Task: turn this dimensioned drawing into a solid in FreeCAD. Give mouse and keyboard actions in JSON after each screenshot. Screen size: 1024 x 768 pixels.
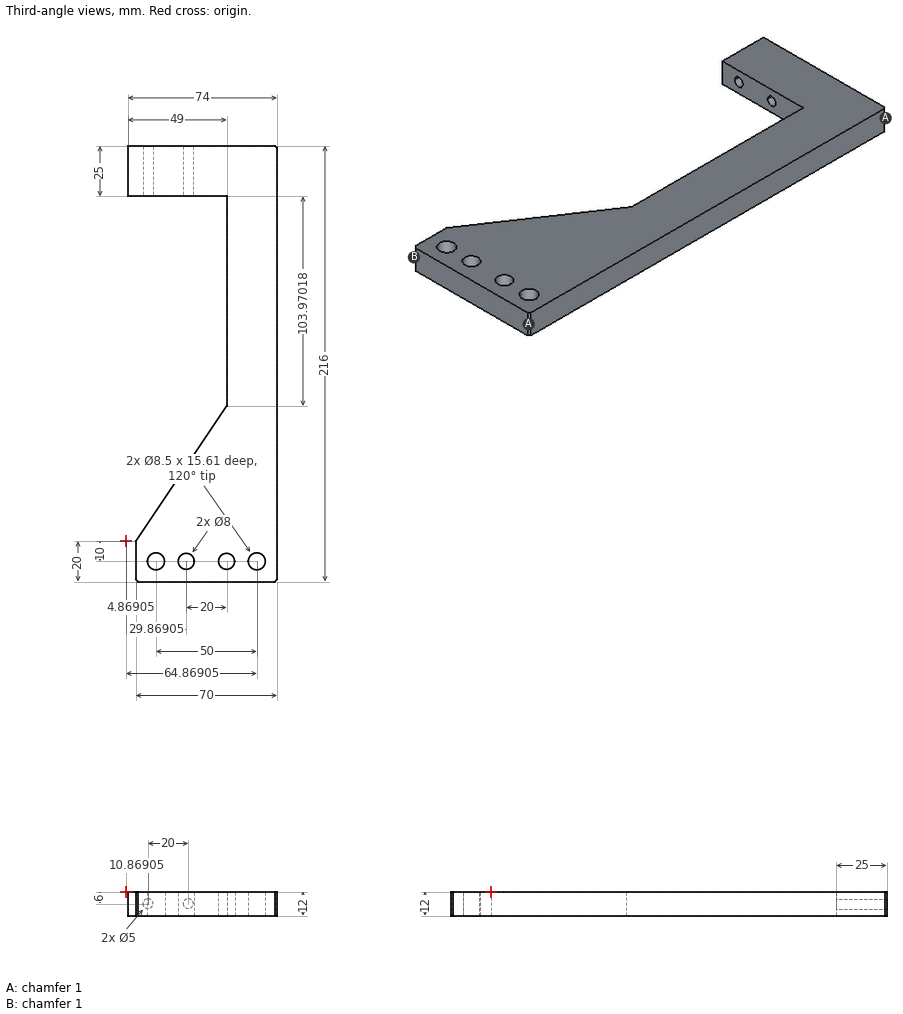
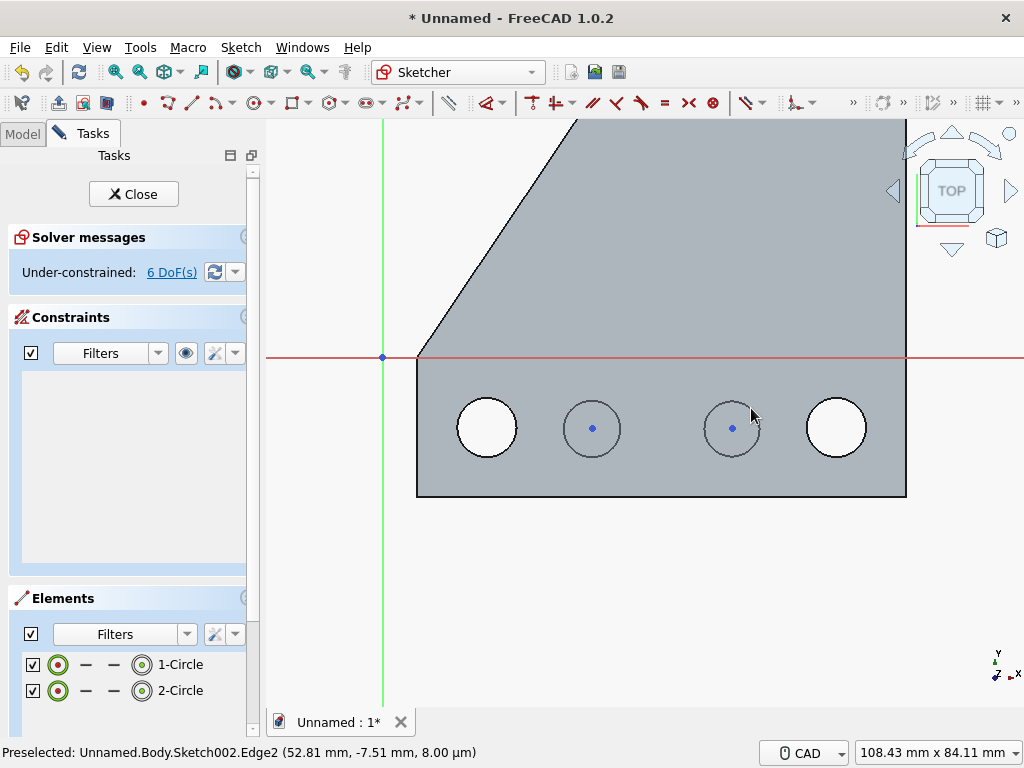
{"action": "left_click", "coordinate": [612, 409]}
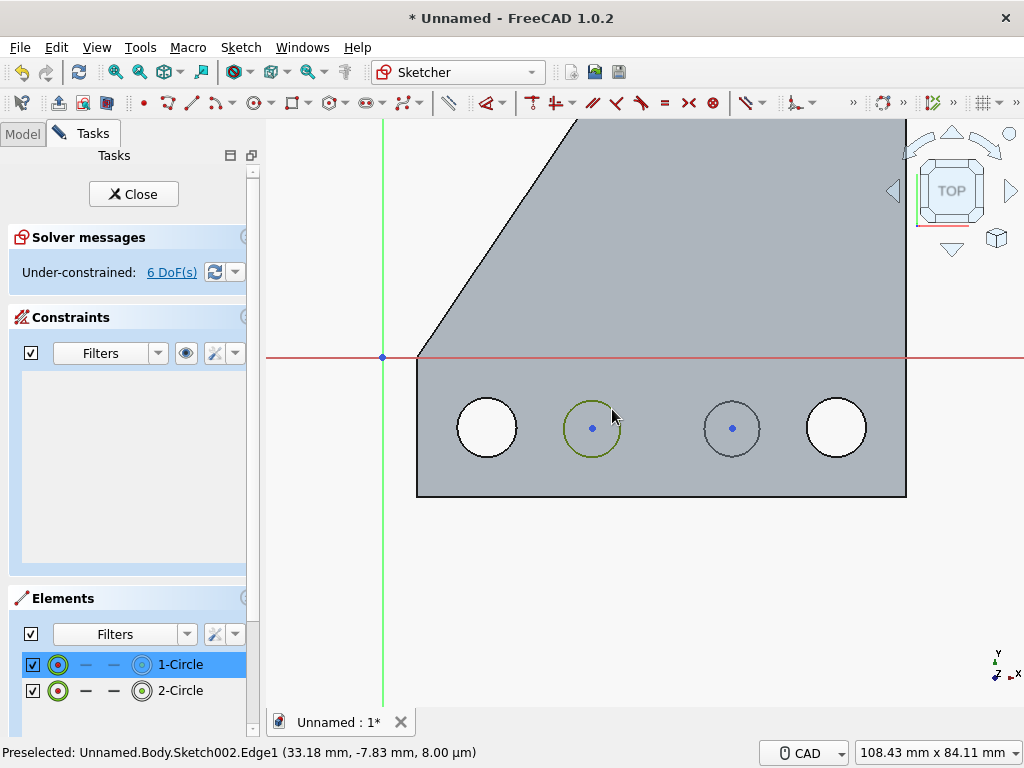
{"action": "left_click", "coordinate": [751, 409]}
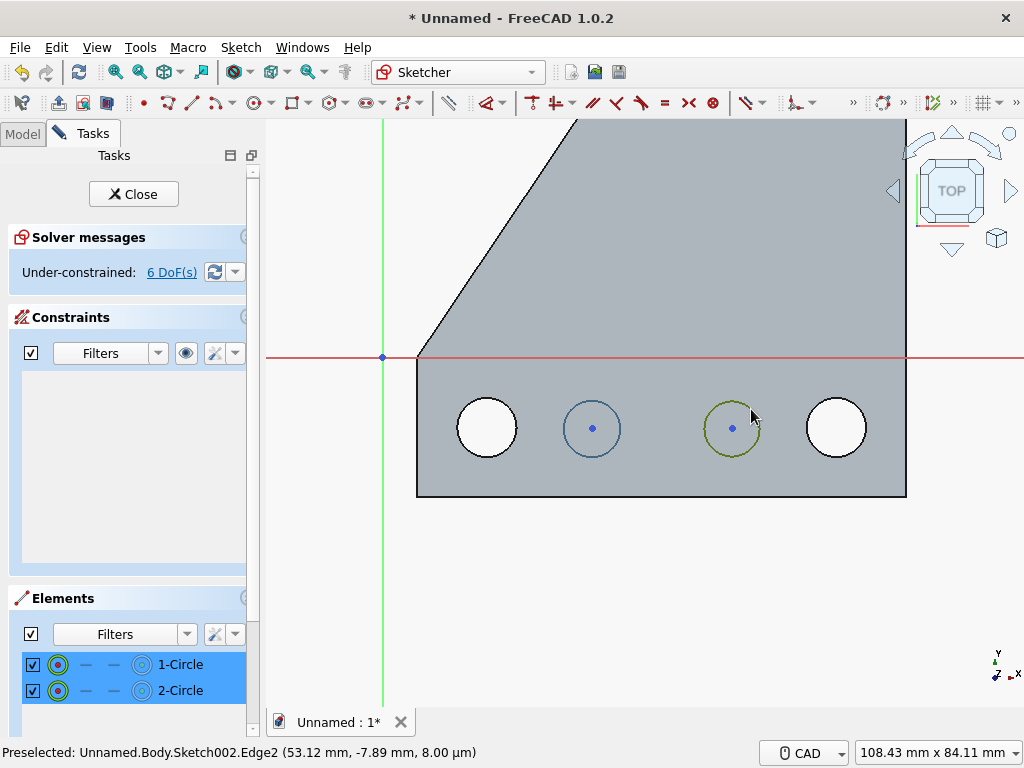
{"action": "left_click", "coordinate": [666, 104]}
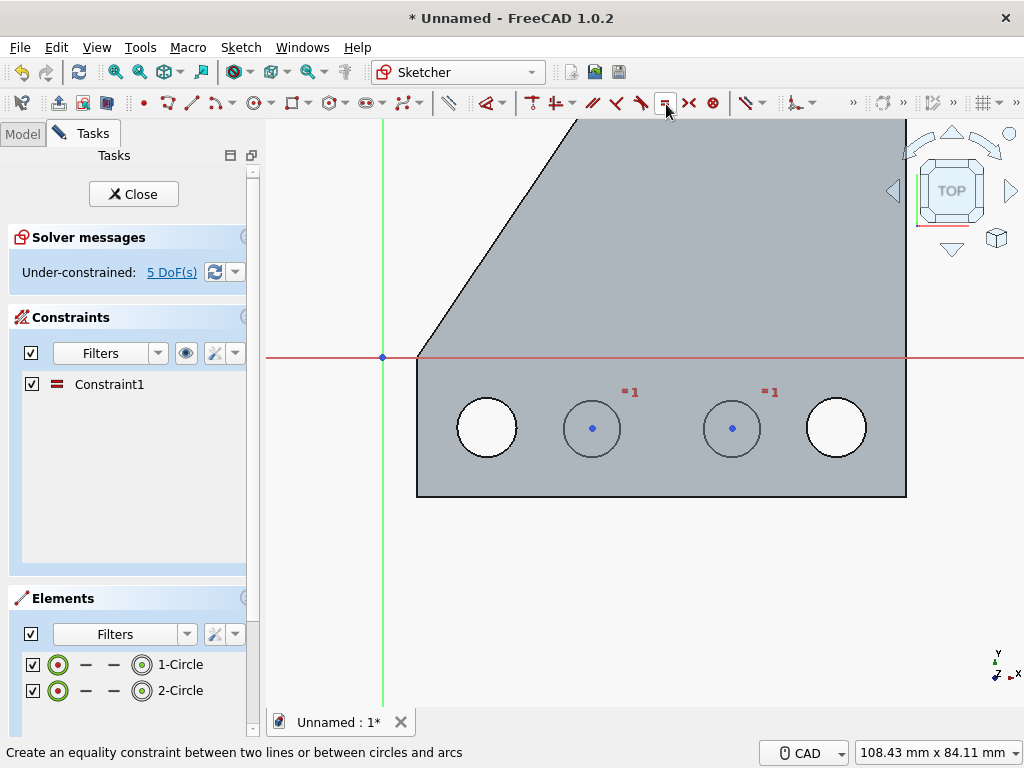
{"action": "key", "text": "d"}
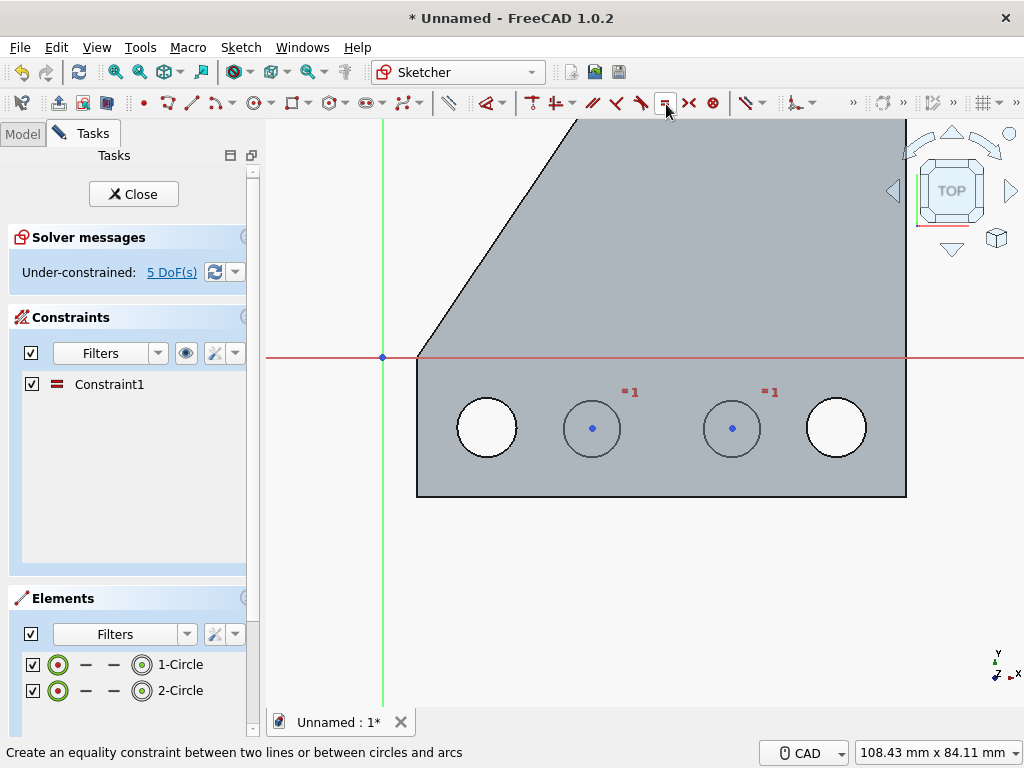
{"action": "left_click", "coordinate": [612, 409]}
{"action": "left_click", "coordinate": [635, 386]}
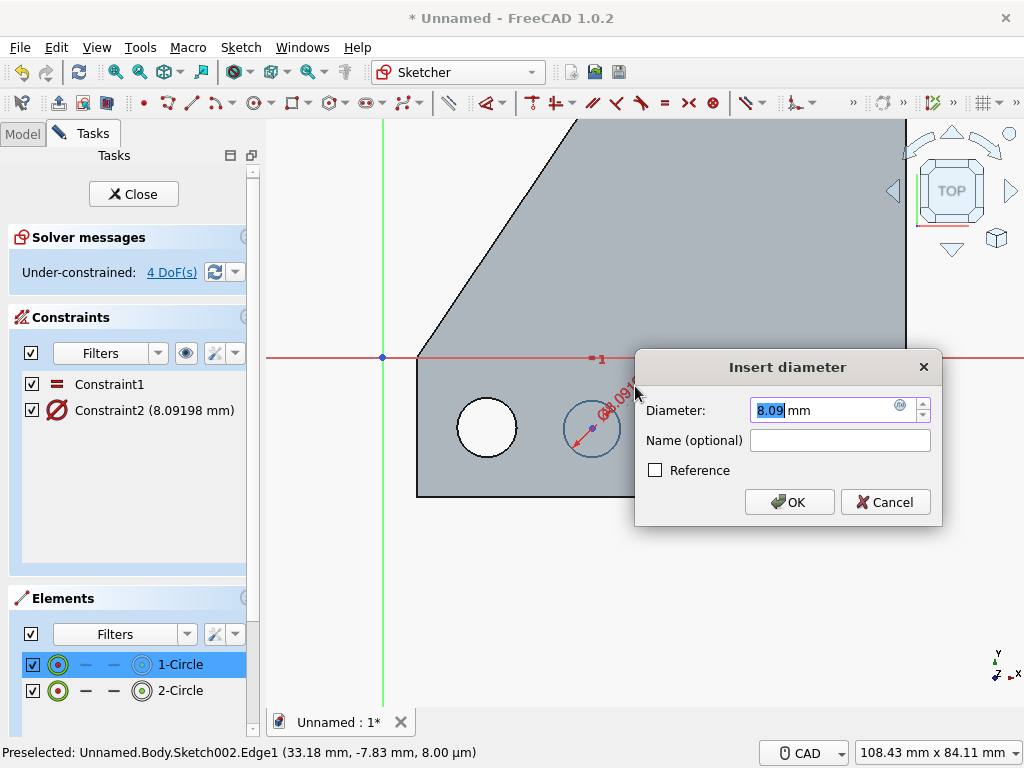
{"action": "type", "text": "8"}
{"action": "key", "text": "Return"}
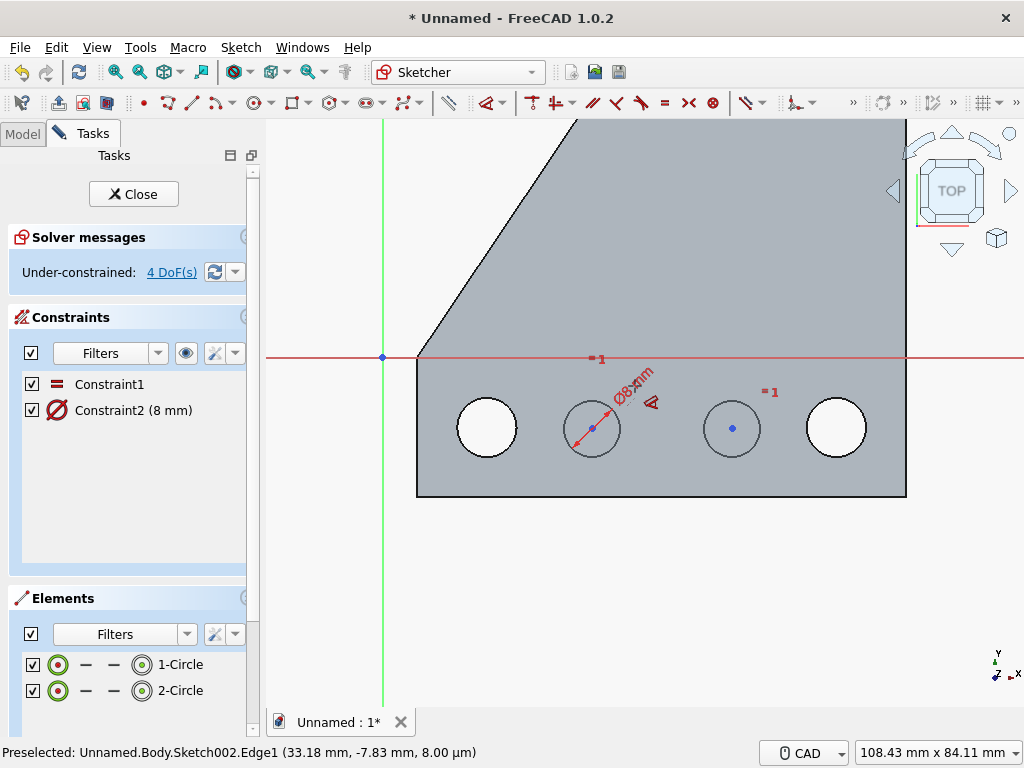
{"action": "left_click", "coordinate": [592, 429]}
{"action": "left_click", "coordinate": [349, 393]}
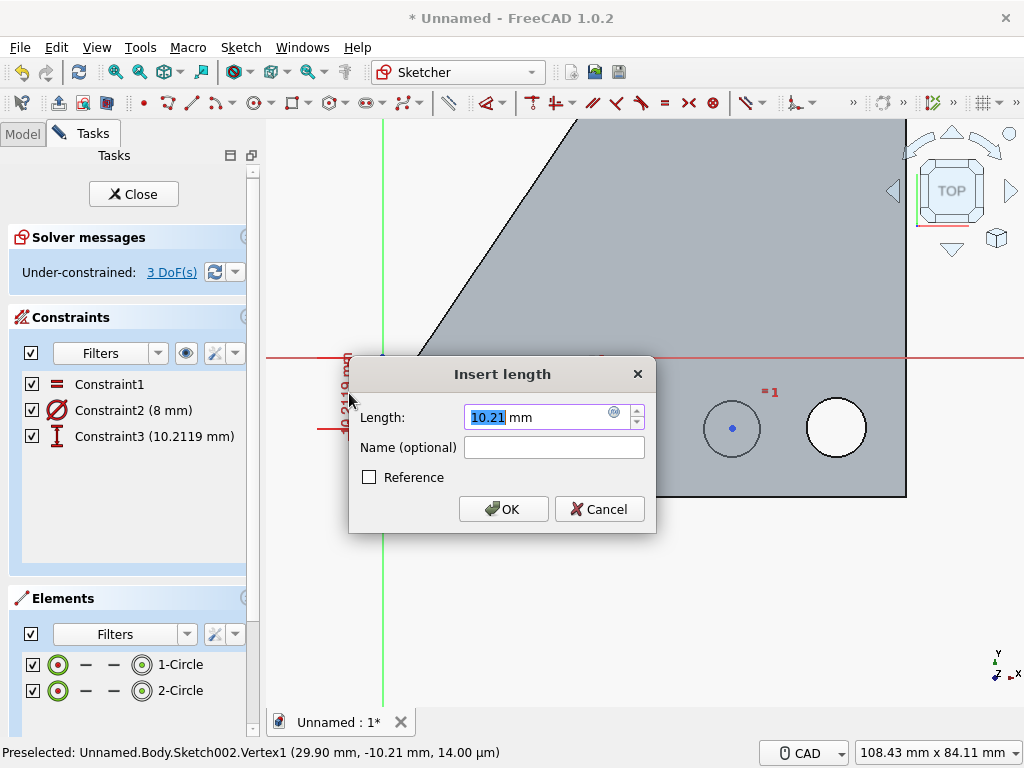
{"action": "type", "text": "10"}
{"action": "key", "text": "Return"}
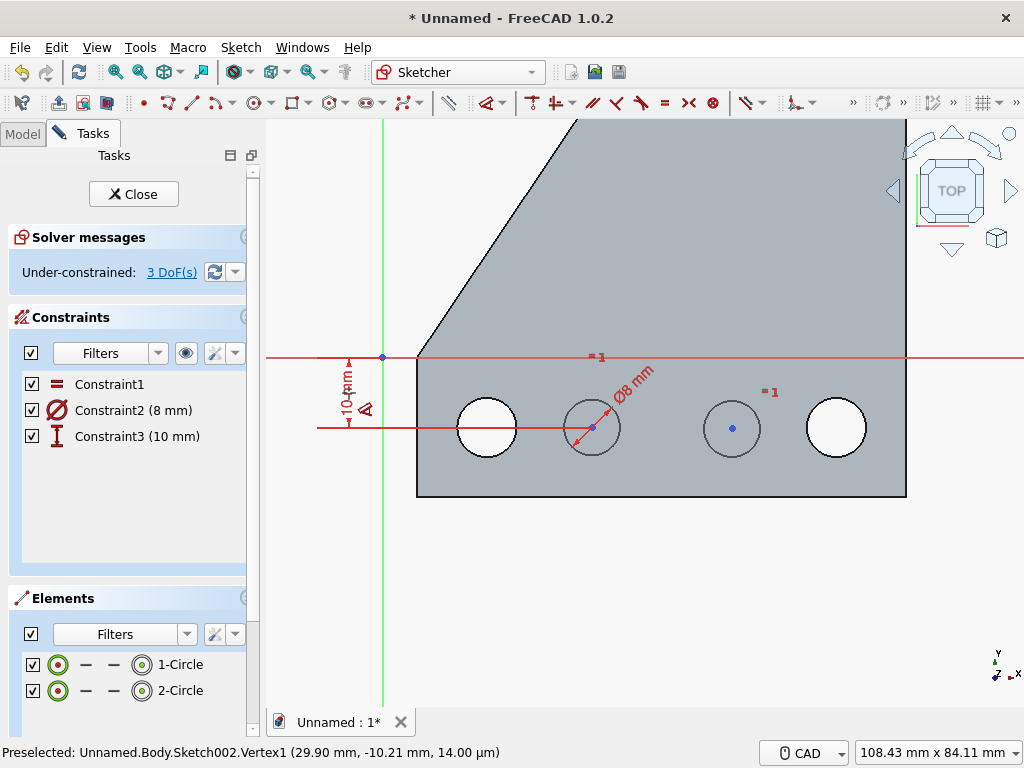
{"action": "left_click", "coordinate": [732, 429]}
{"action": "left_click", "coordinate": [349, 418]}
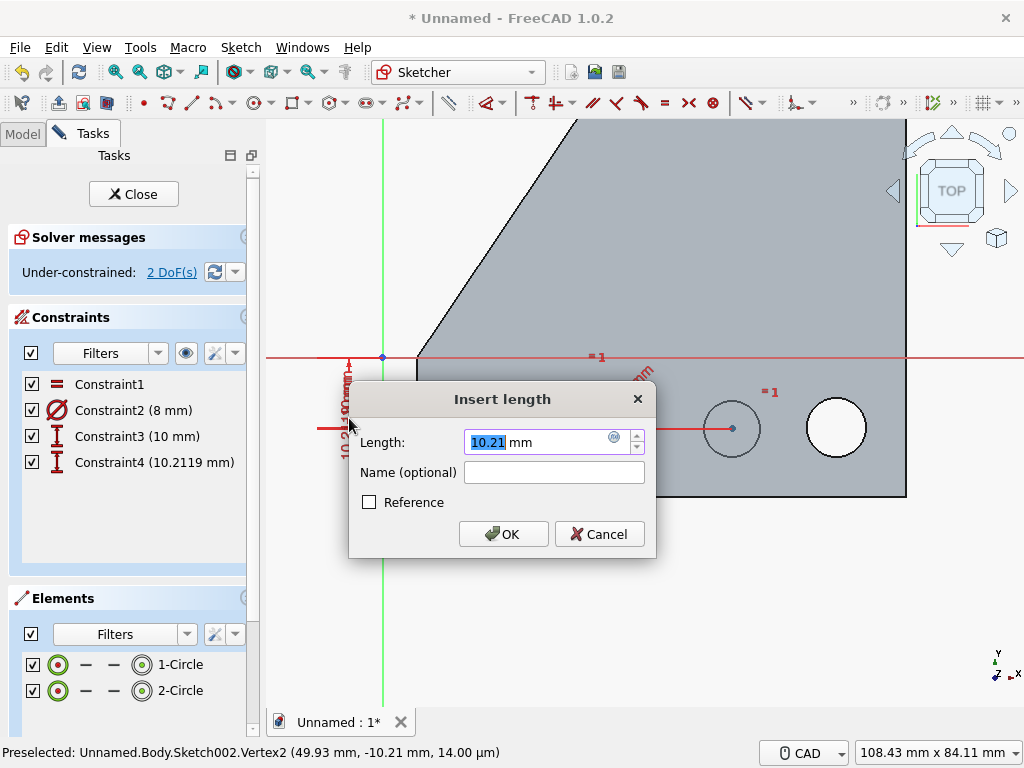
{"action": "type", "text": "10"}
{"action": "key", "text": "Return"}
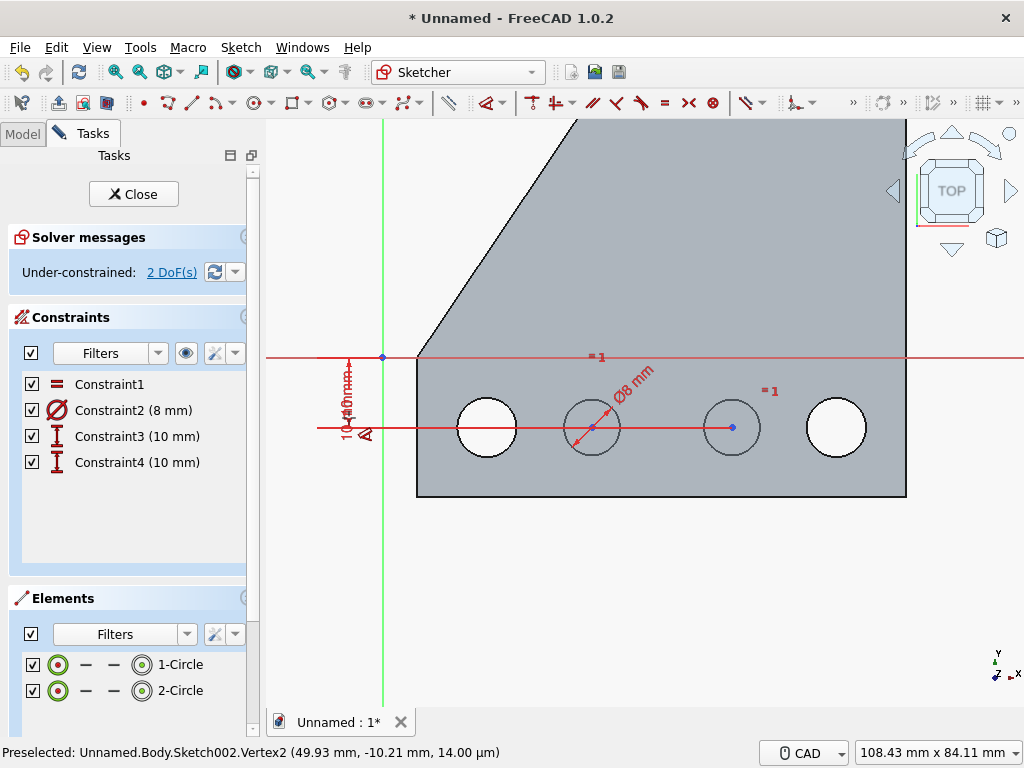
{"action": "left_click", "coordinate": [592, 428]}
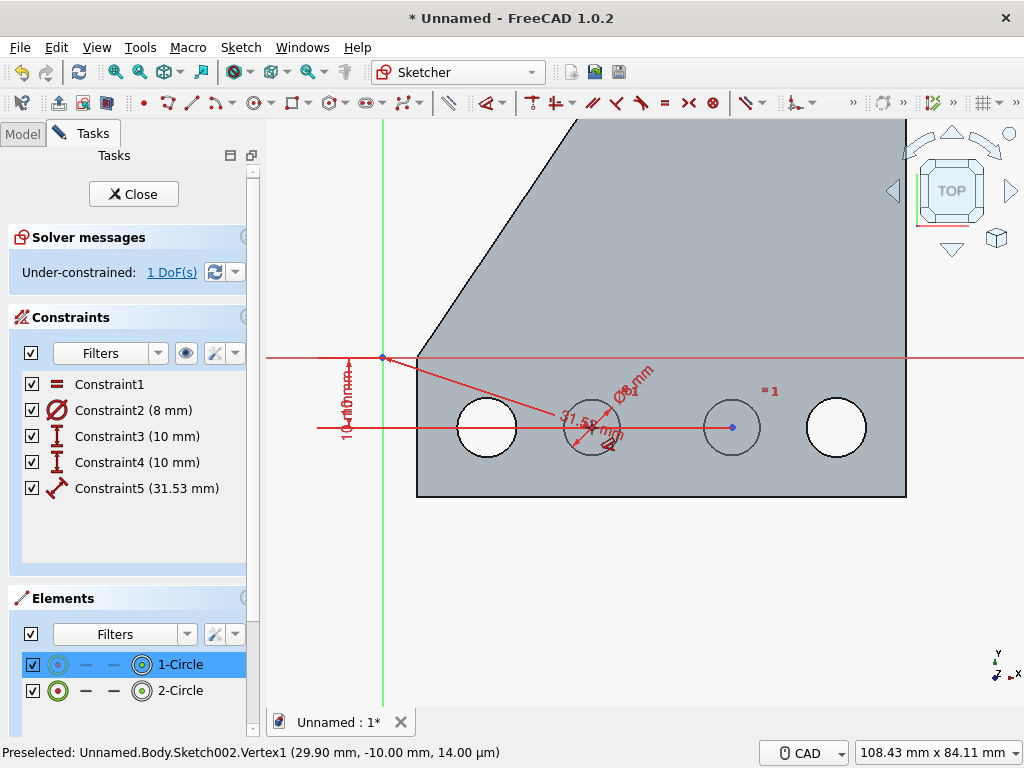
{"action": "left_click", "coordinate": [732, 428]}
{"action": "left_click", "coordinate": [662, 462]}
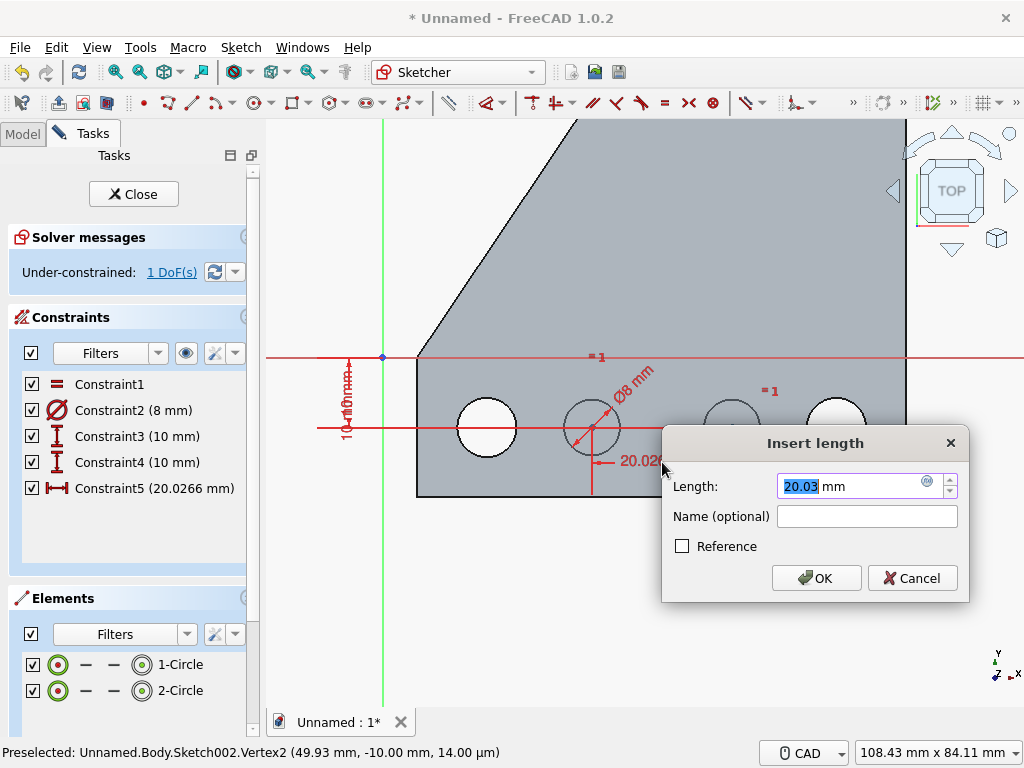
{"action": "type", "text": "20"}
{"action": "key", "text": "Return"}